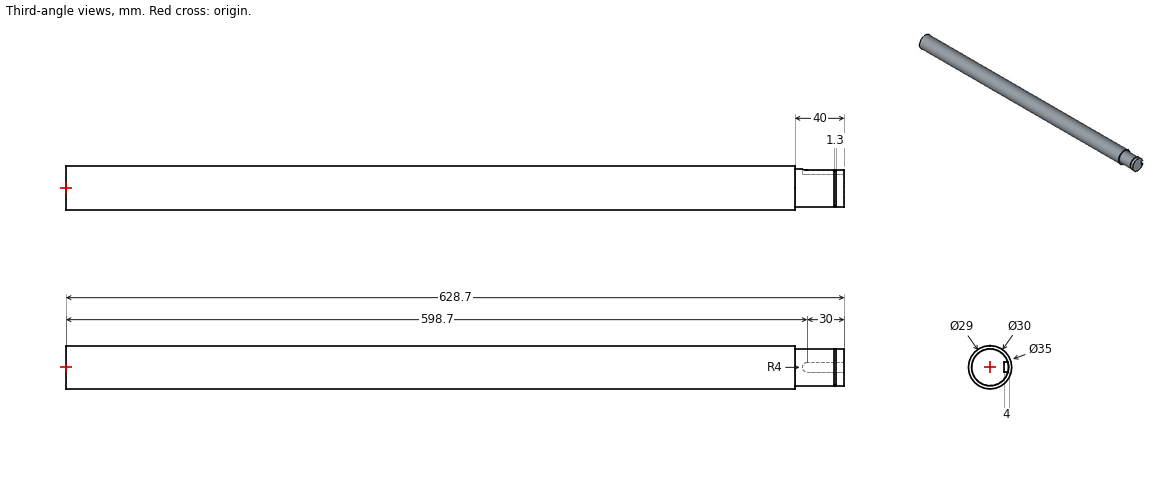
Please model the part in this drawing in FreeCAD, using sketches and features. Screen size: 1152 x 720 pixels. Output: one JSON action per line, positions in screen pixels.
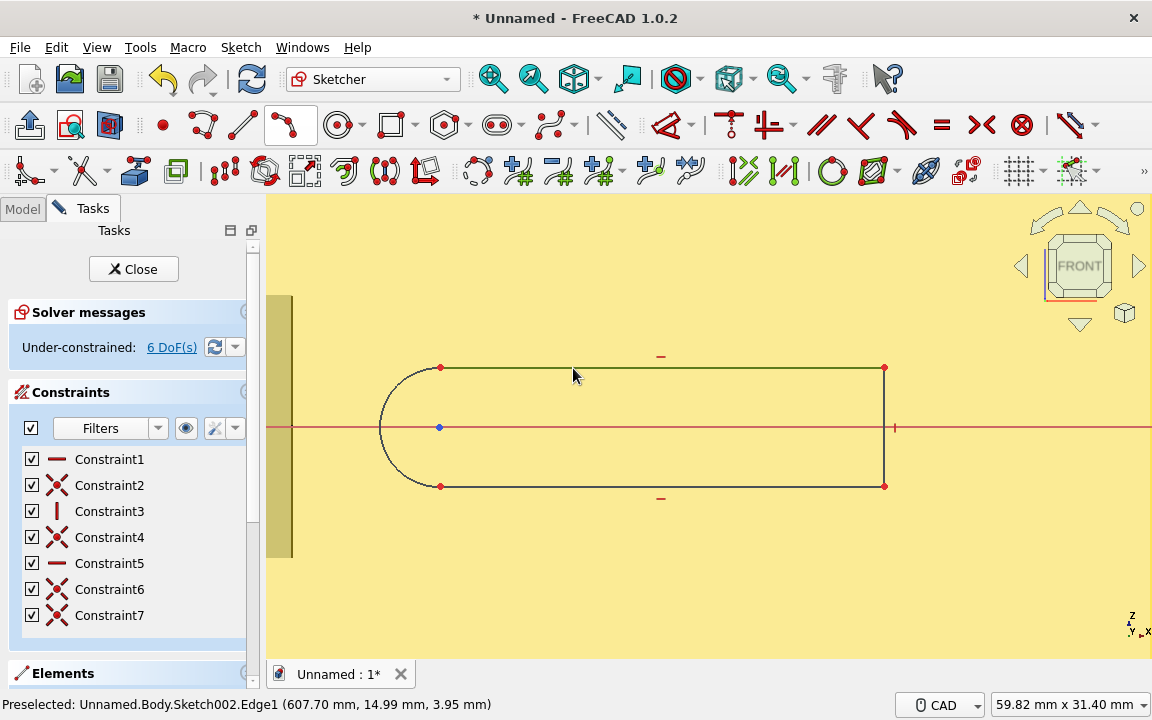
{"action": "left_click", "coordinate": [392, 392]}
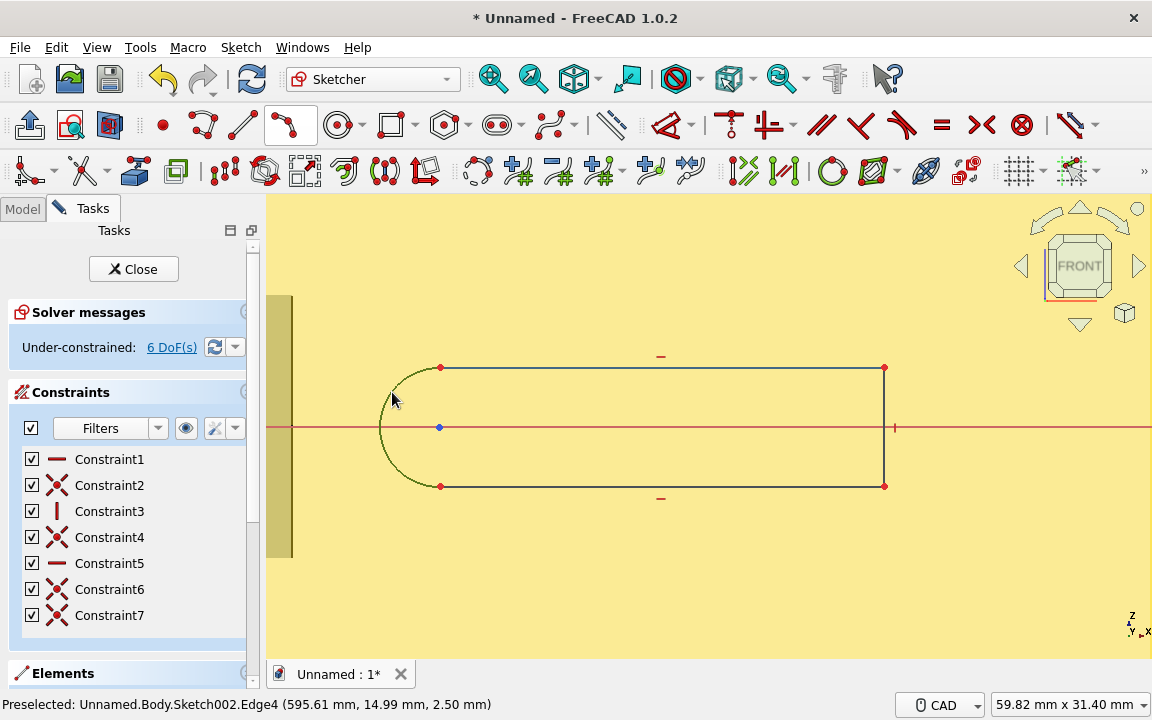
{"action": "left_click", "coordinate": [902, 126]}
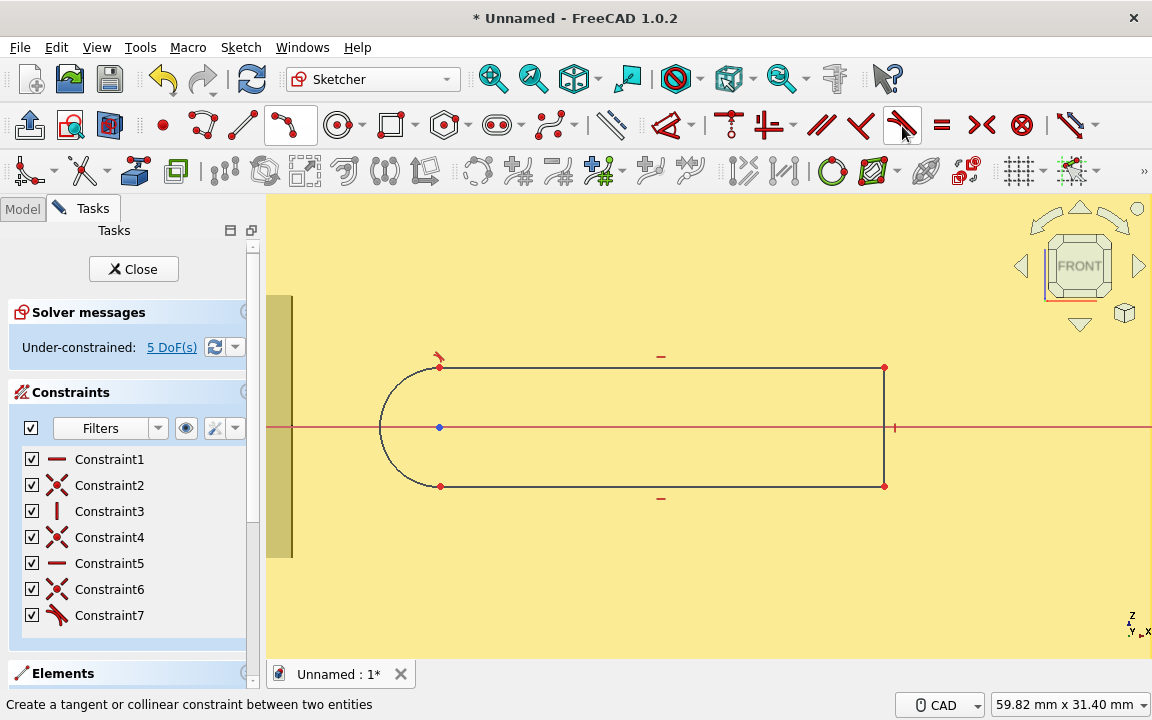
{"action": "left_click", "coordinate": [751, 487]}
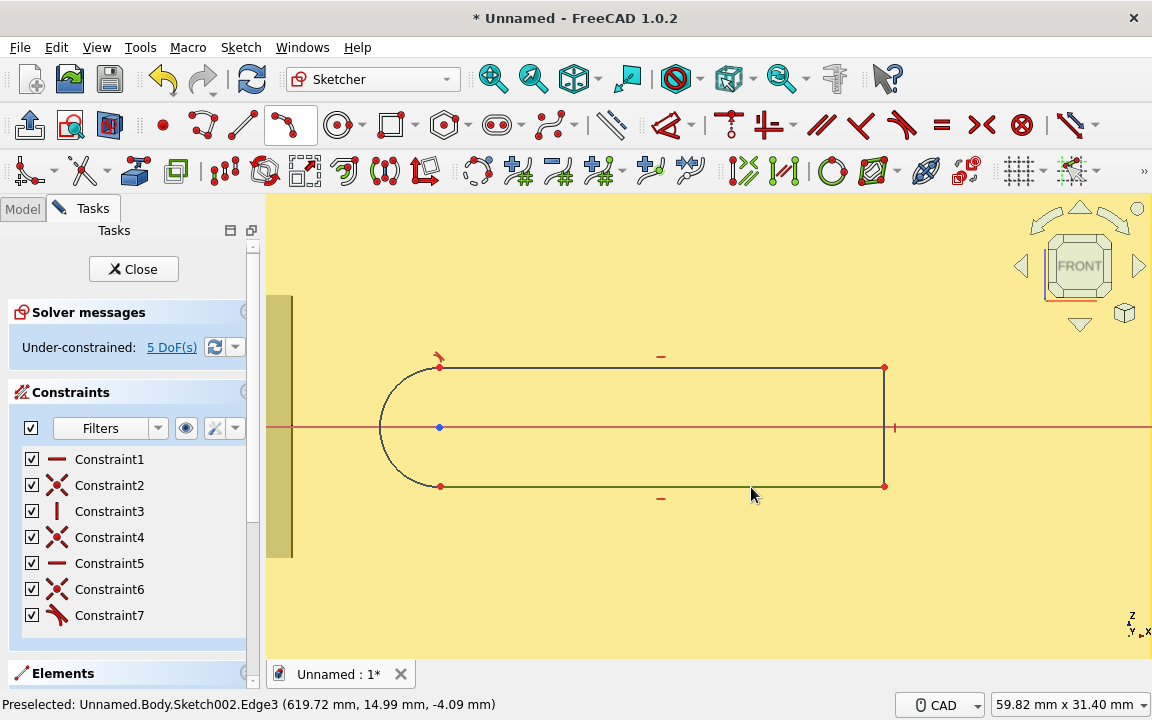
{"action": "left_click", "coordinate": [391, 393]}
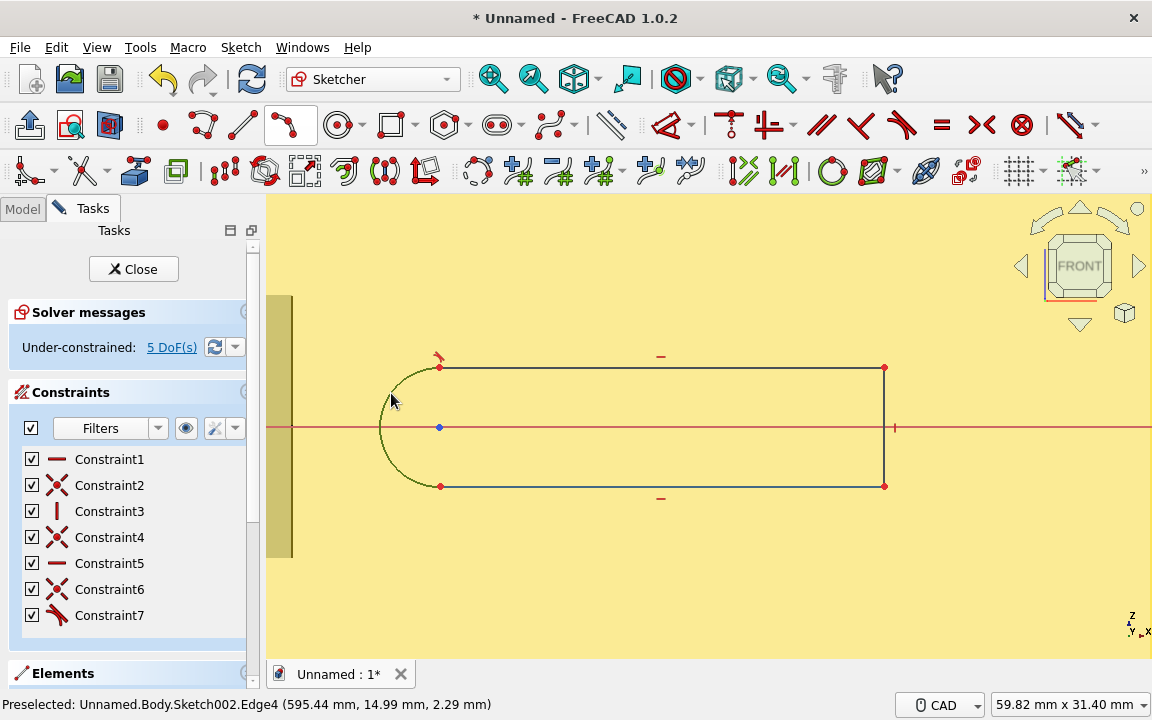
{"action": "left_click", "coordinate": [902, 126]}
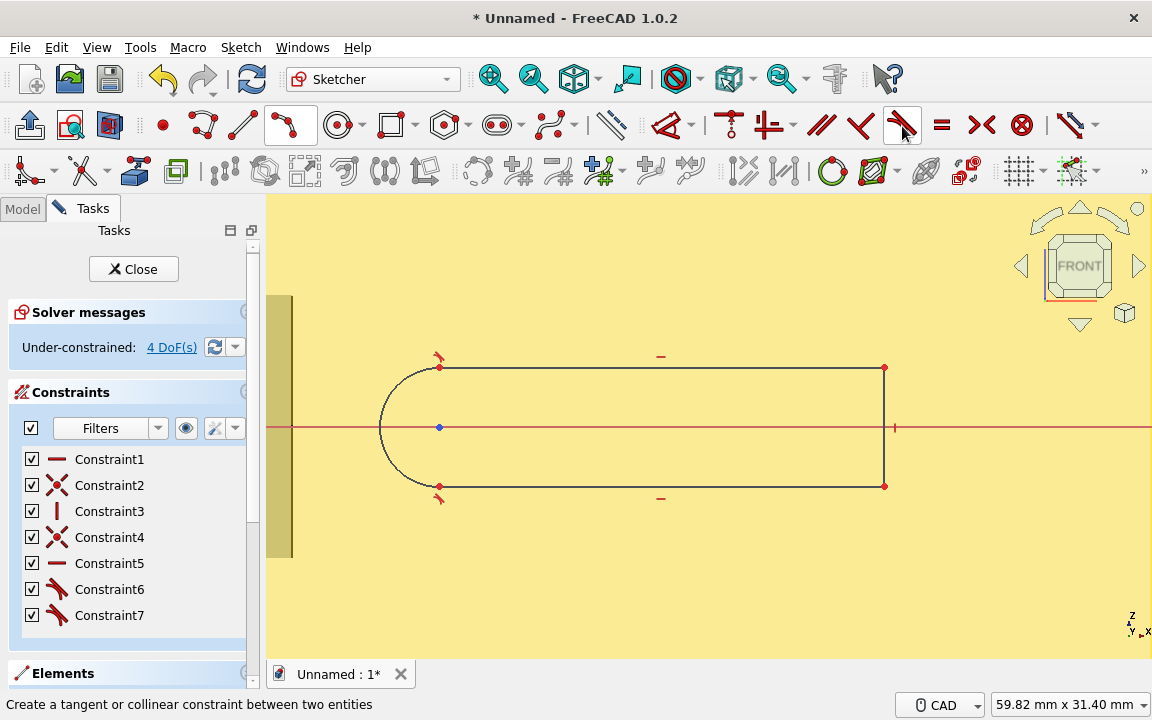
{"action": "left_click", "coordinate": [440, 427]}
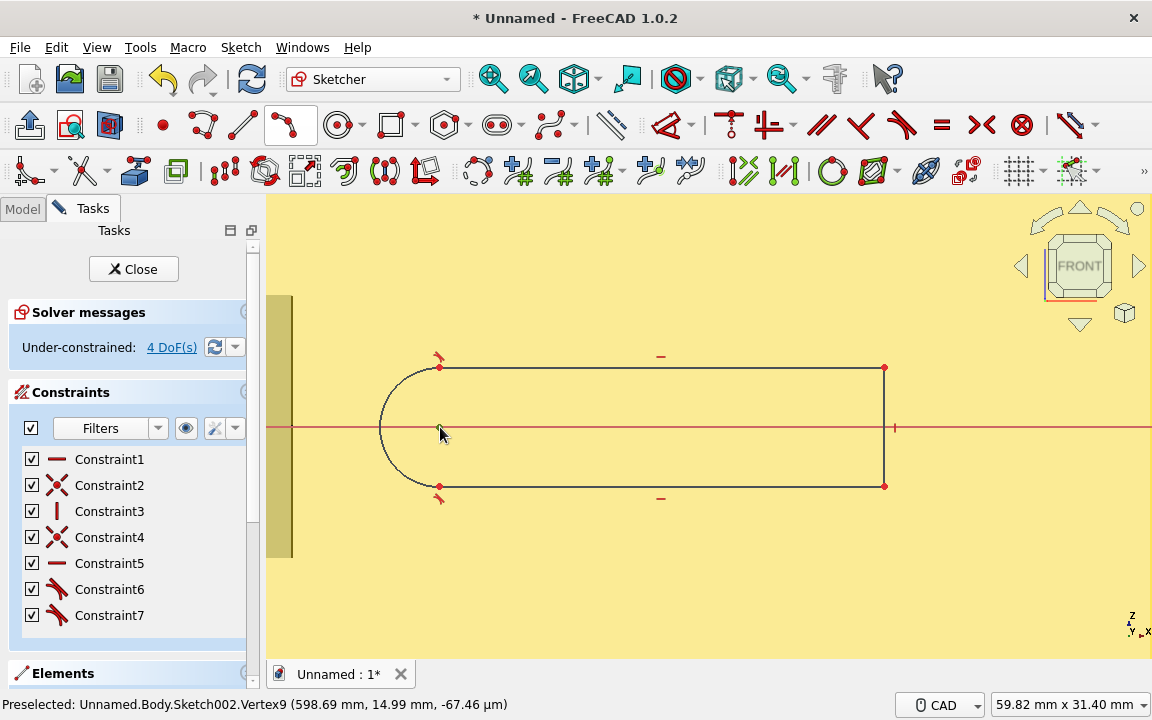
{"action": "left_click", "coordinate": [344, 427]}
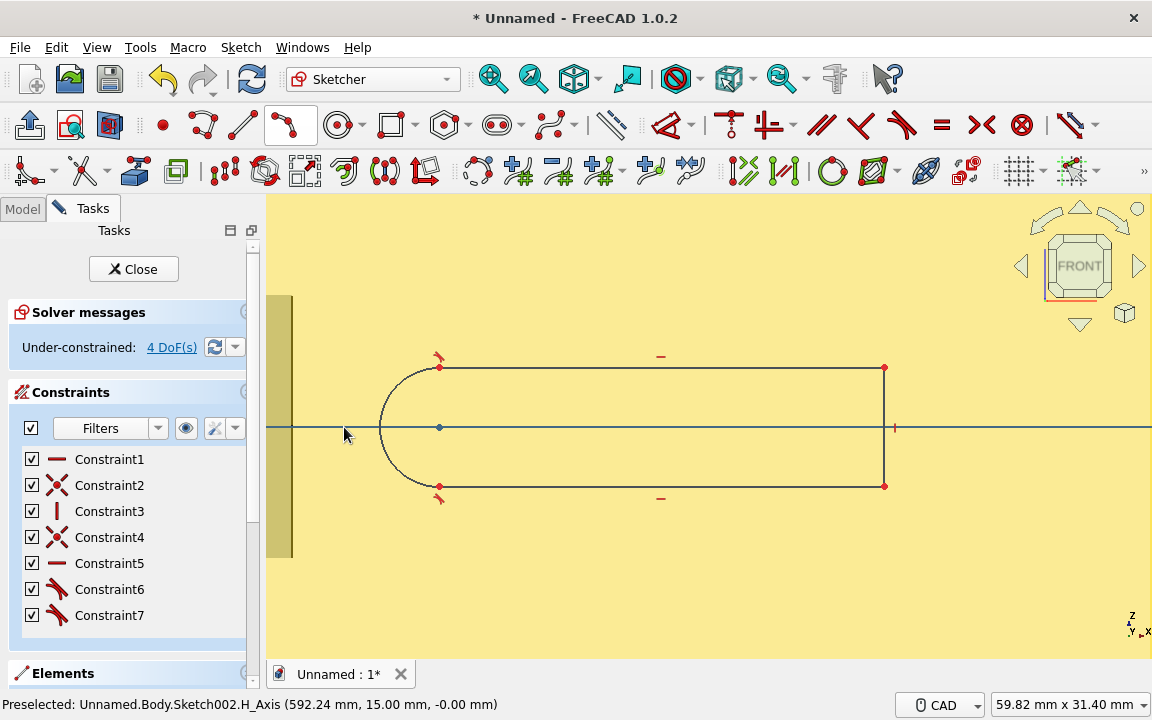
{"action": "left_click", "coordinate": [730, 126]}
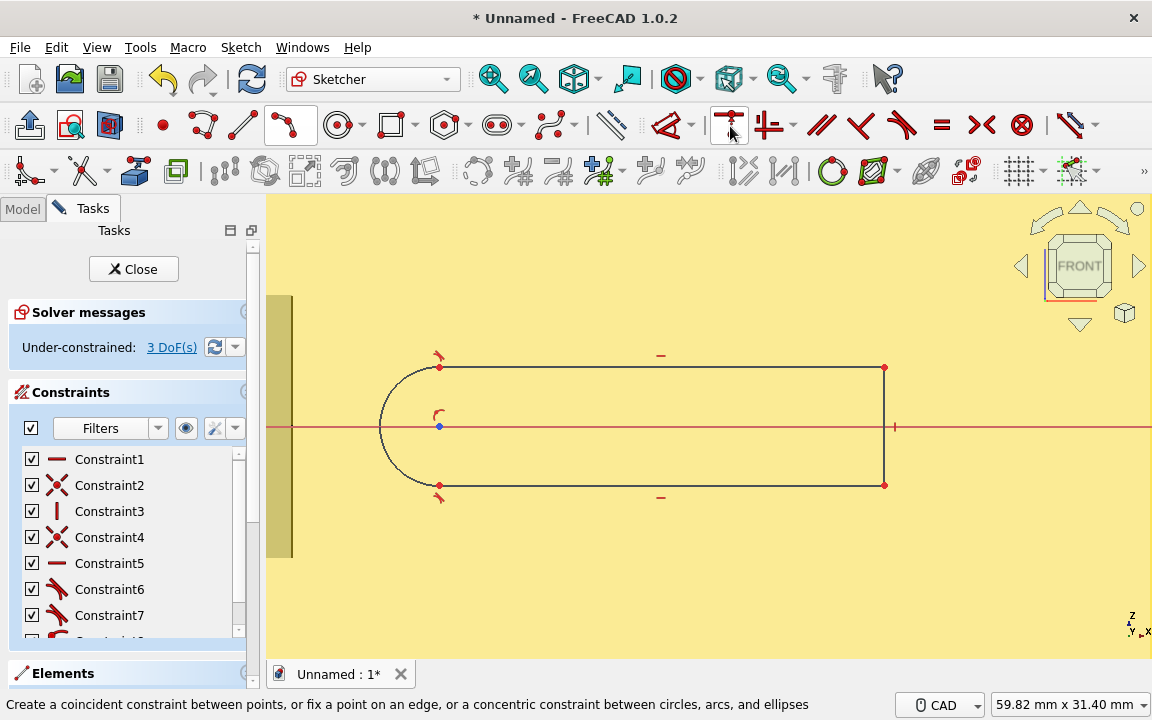
{"action": "left_click", "coordinate": [666, 126]}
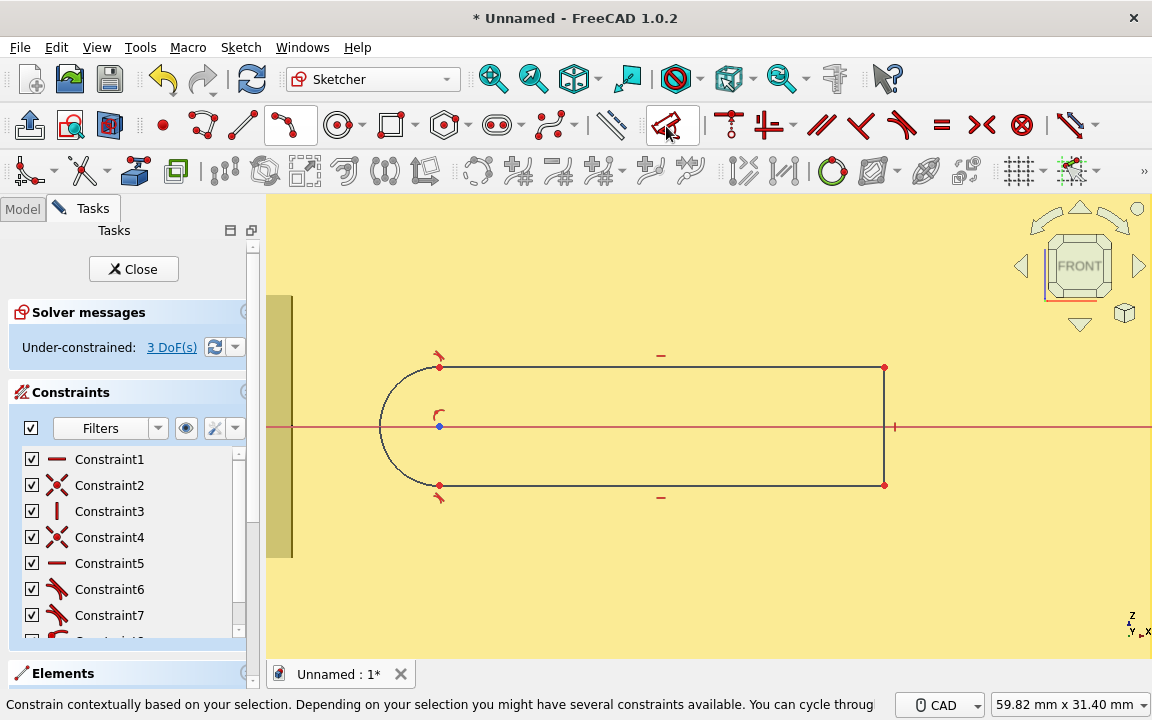
{"action": "left_click", "coordinate": [391, 392]}
{"action": "left_click", "coordinate": [365, 373]}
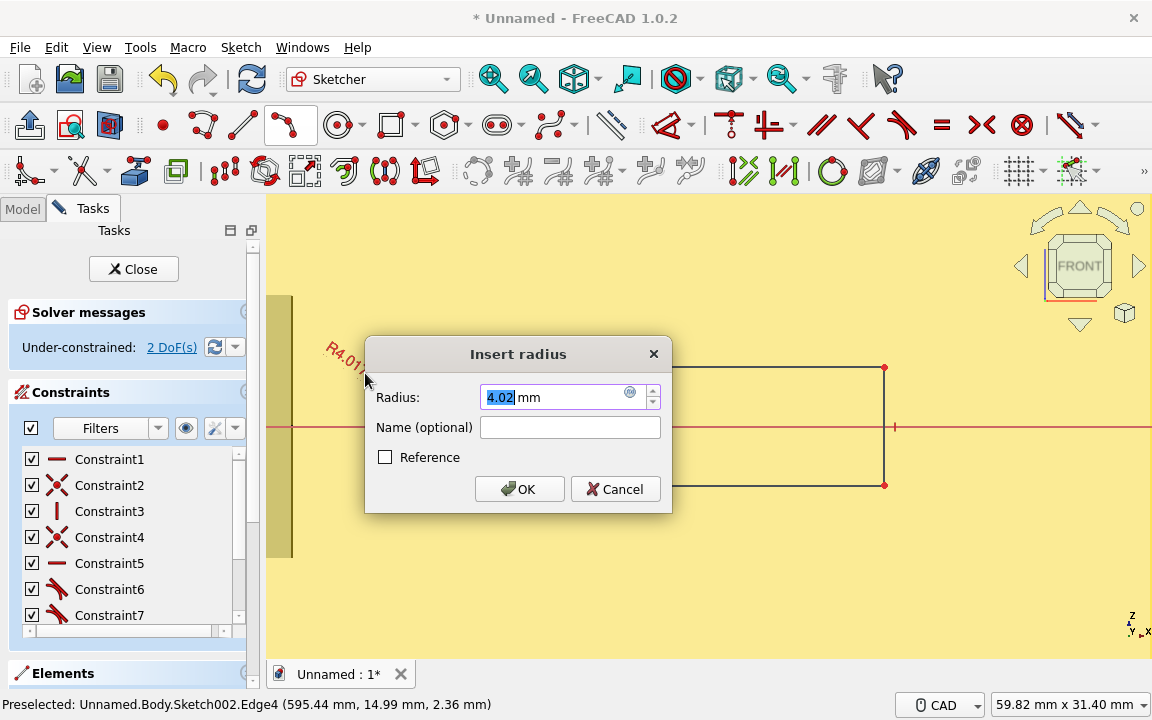
{"action": "type", "text": "4"}
{"action": "key", "text": "Return"}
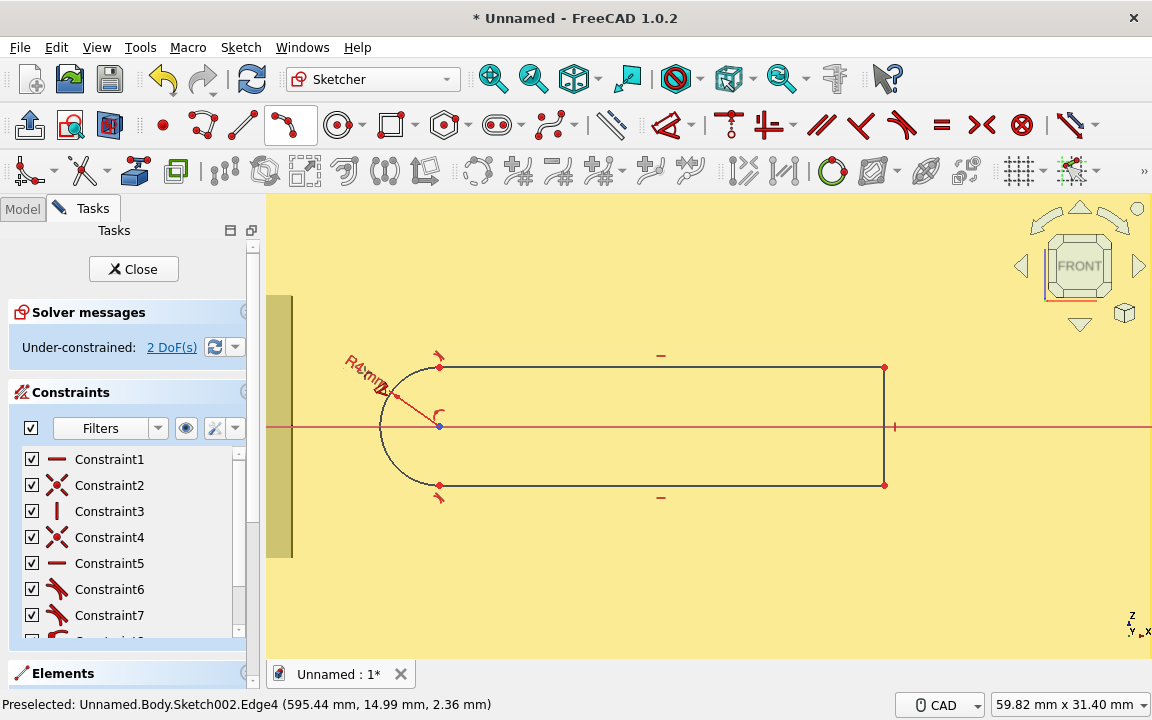
{"action": "left_click", "coordinate": [573, 367]}
{"action": "left_click", "coordinate": [662, 333]}